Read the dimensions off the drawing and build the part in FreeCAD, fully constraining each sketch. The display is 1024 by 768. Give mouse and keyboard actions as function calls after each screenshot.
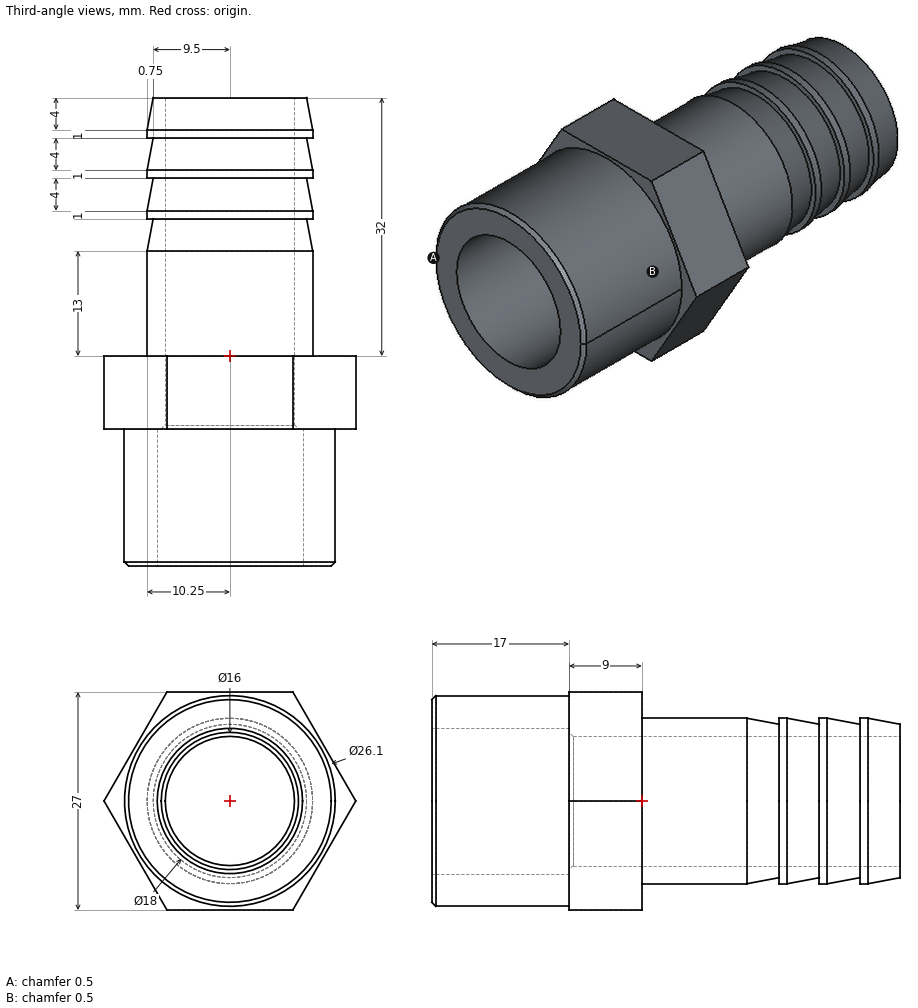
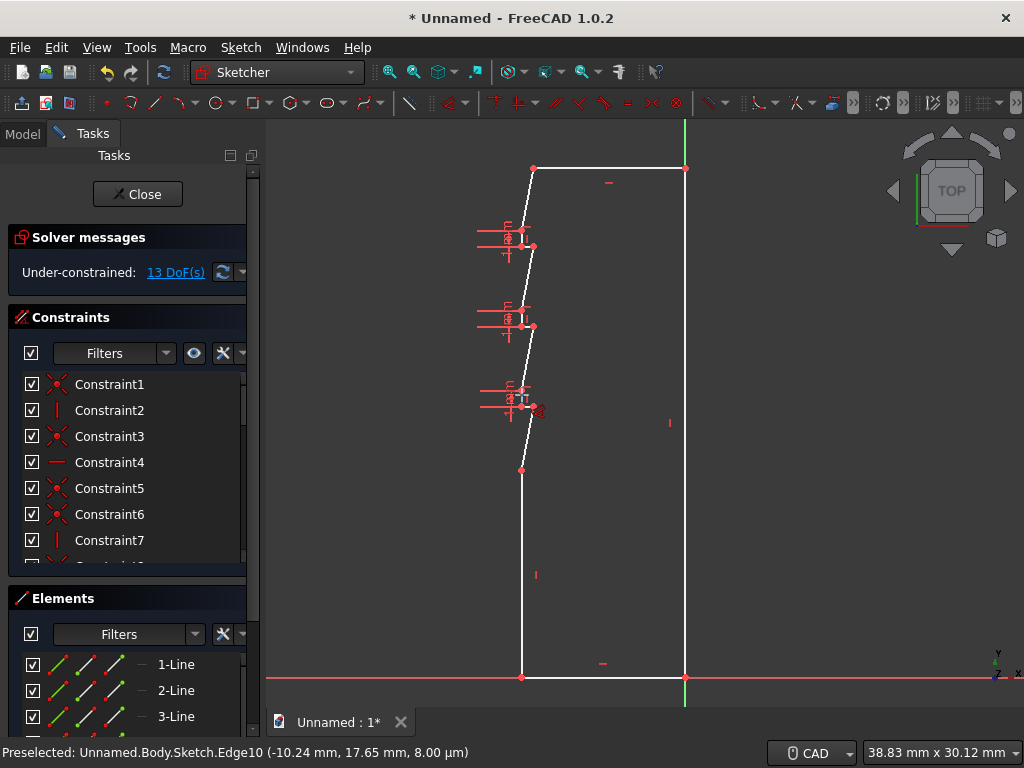
click(631, 482)
click(665, 414)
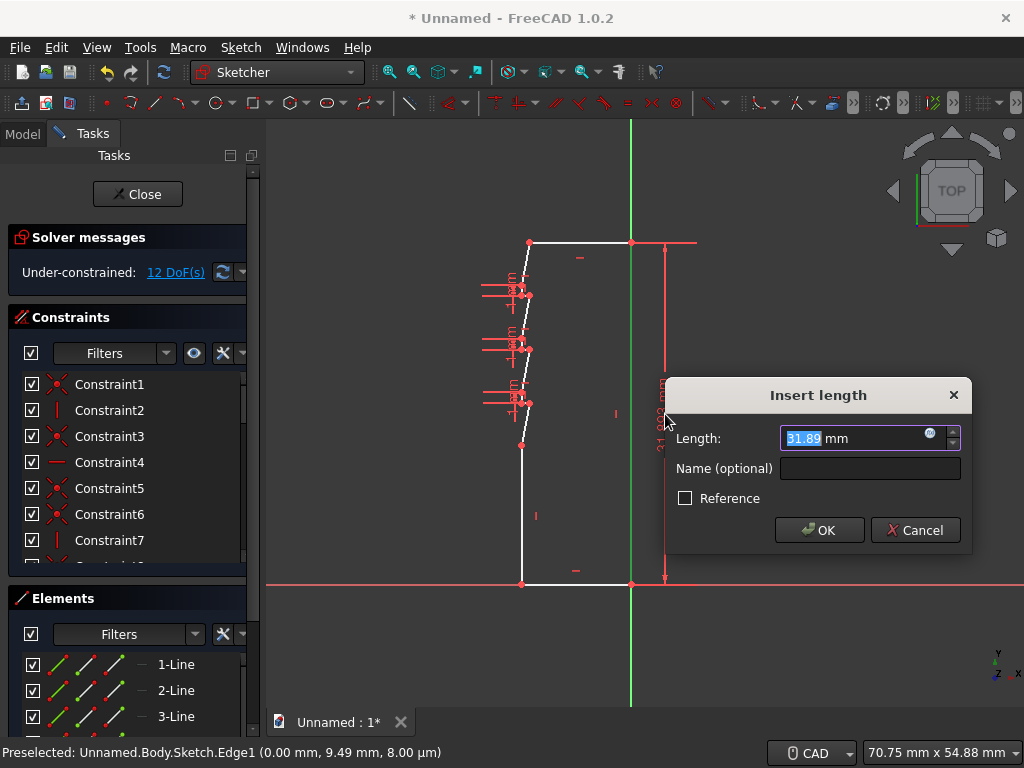
text(32)
key(Return)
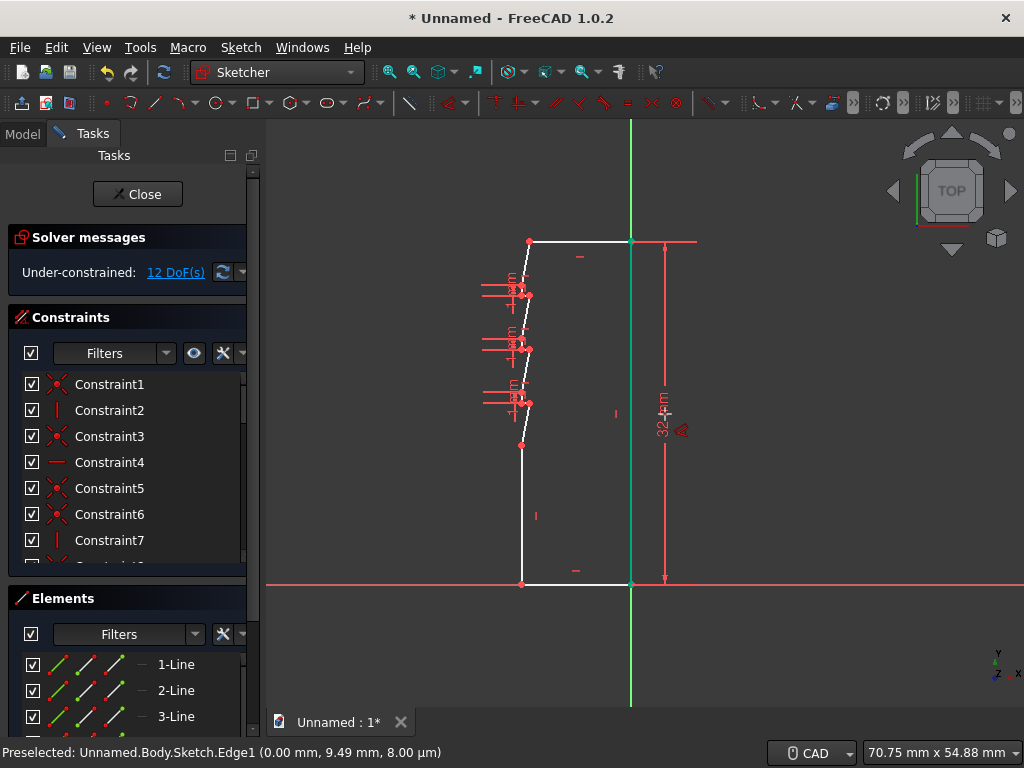
click(522, 487)
click(488, 515)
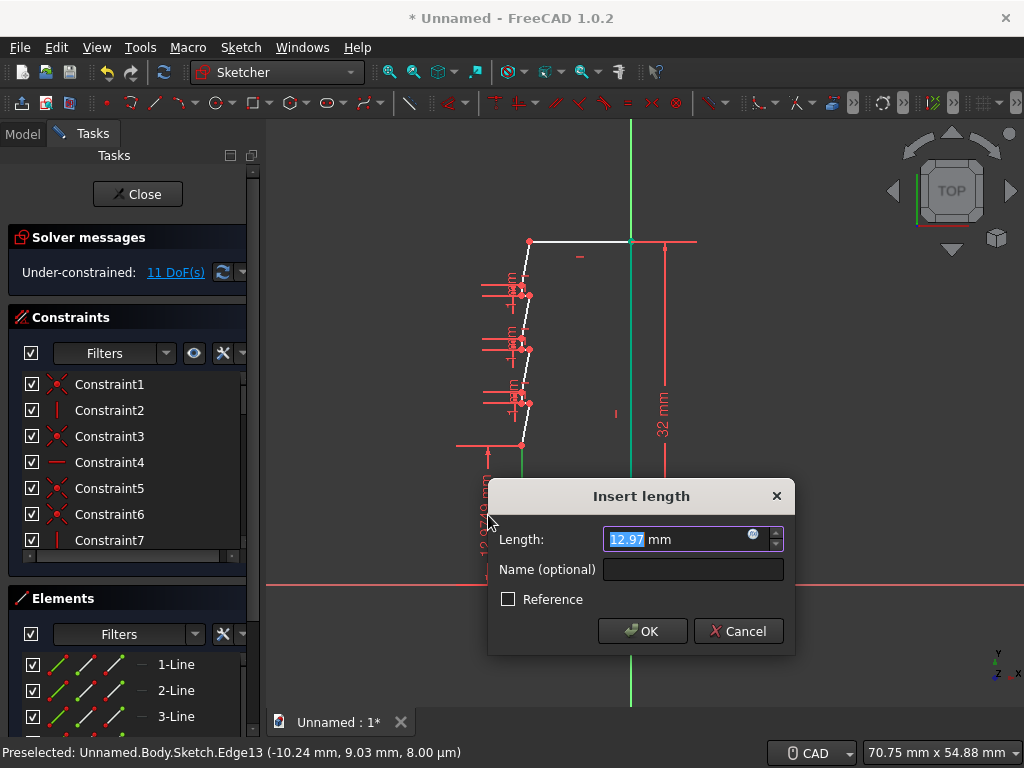
text(13)
key(Return)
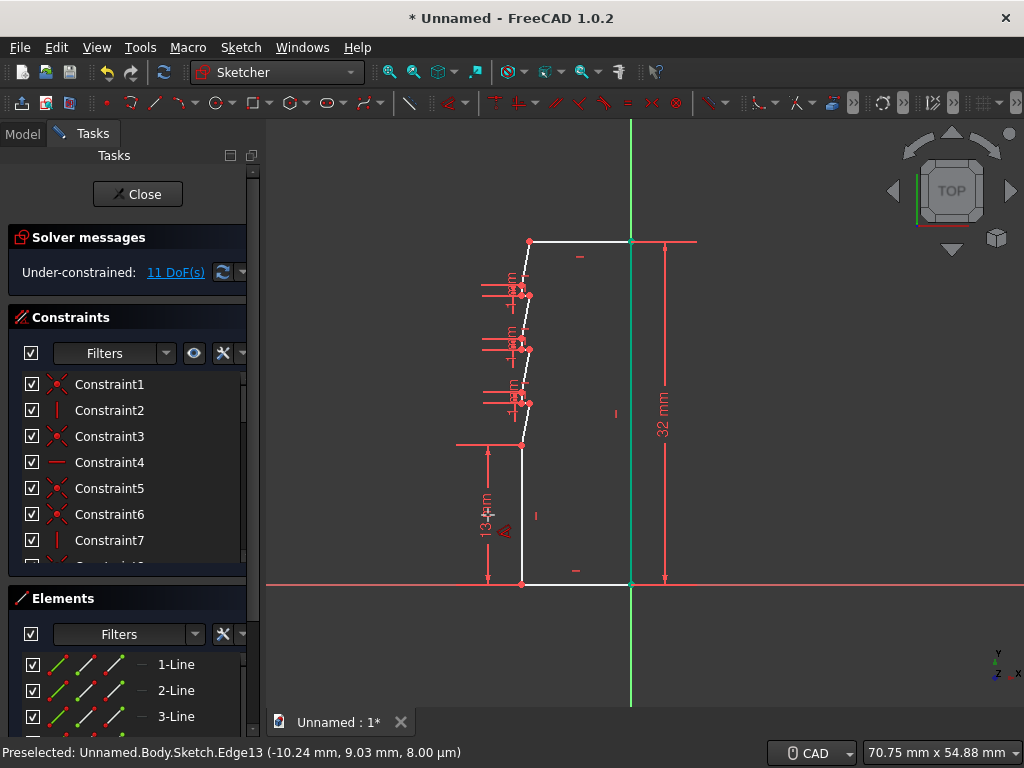
click(527, 255)
click(488, 263)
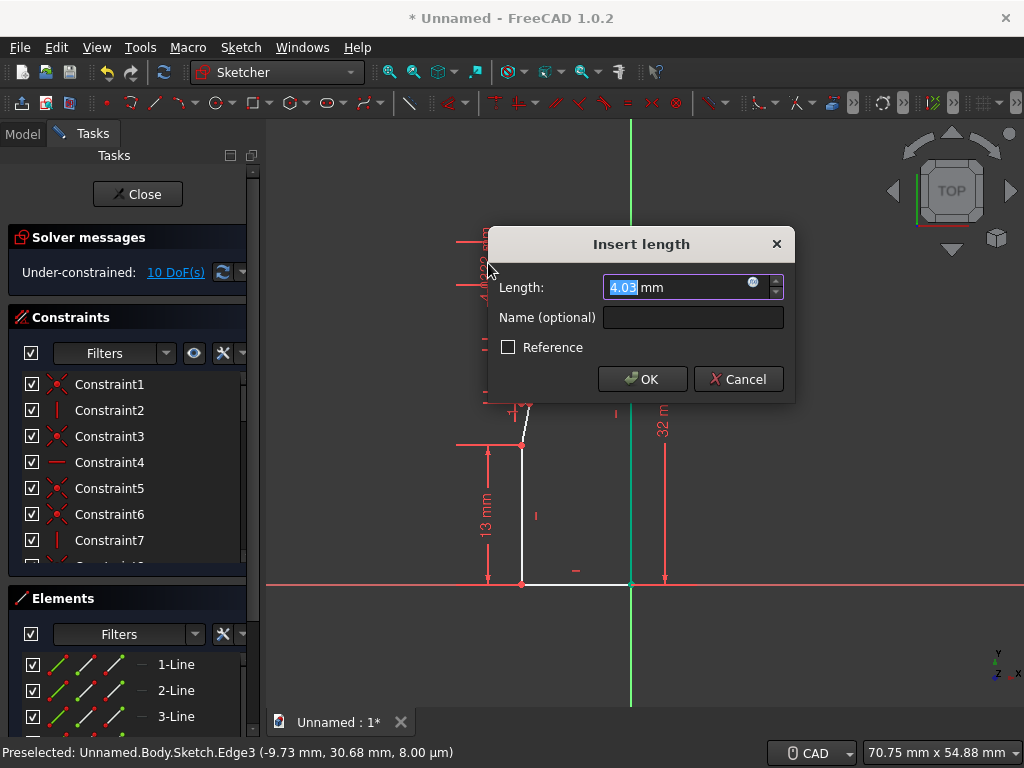
text(4)
key(Return)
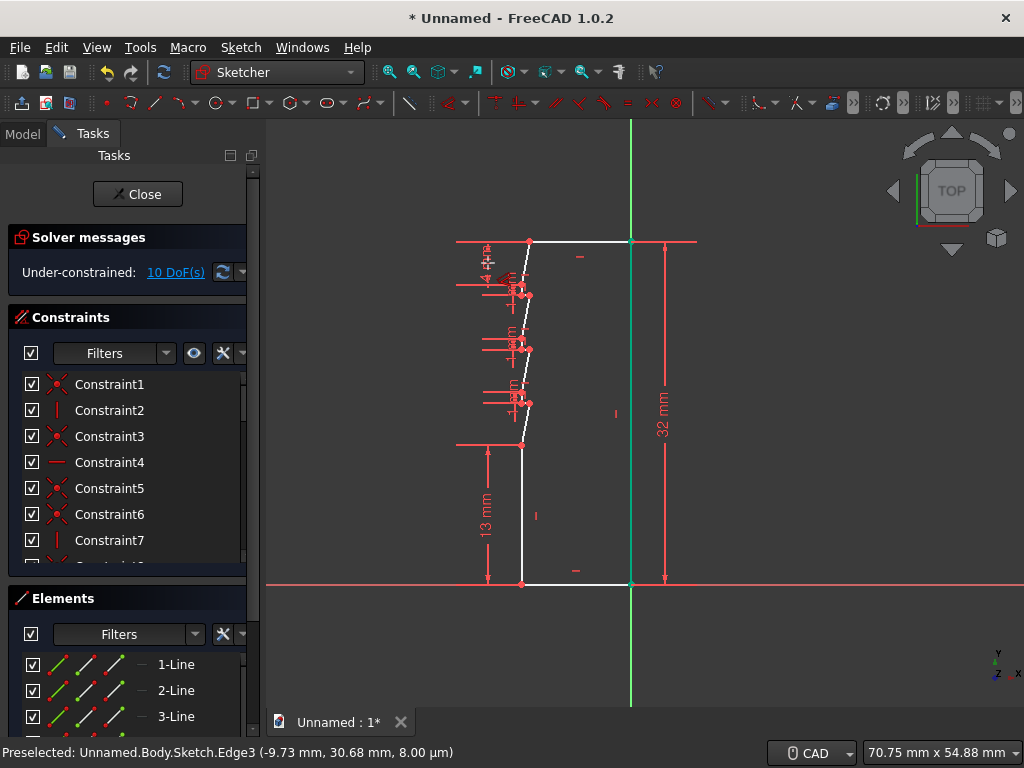
click(527, 308)
click(488, 317)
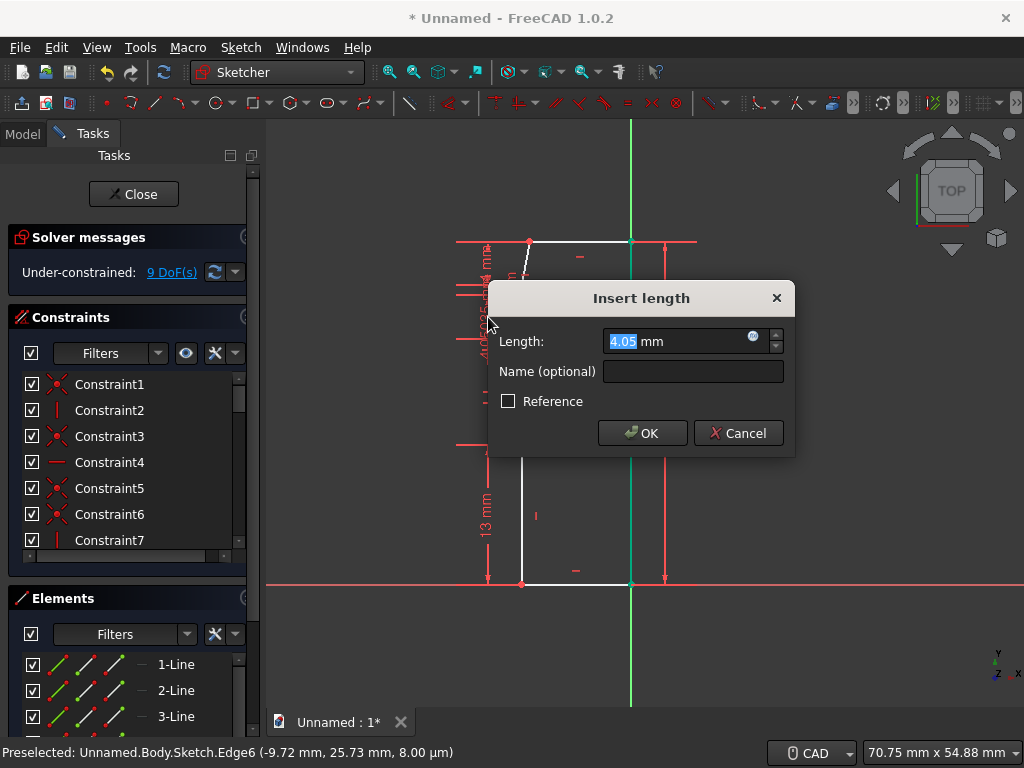
text(4)
key(Return)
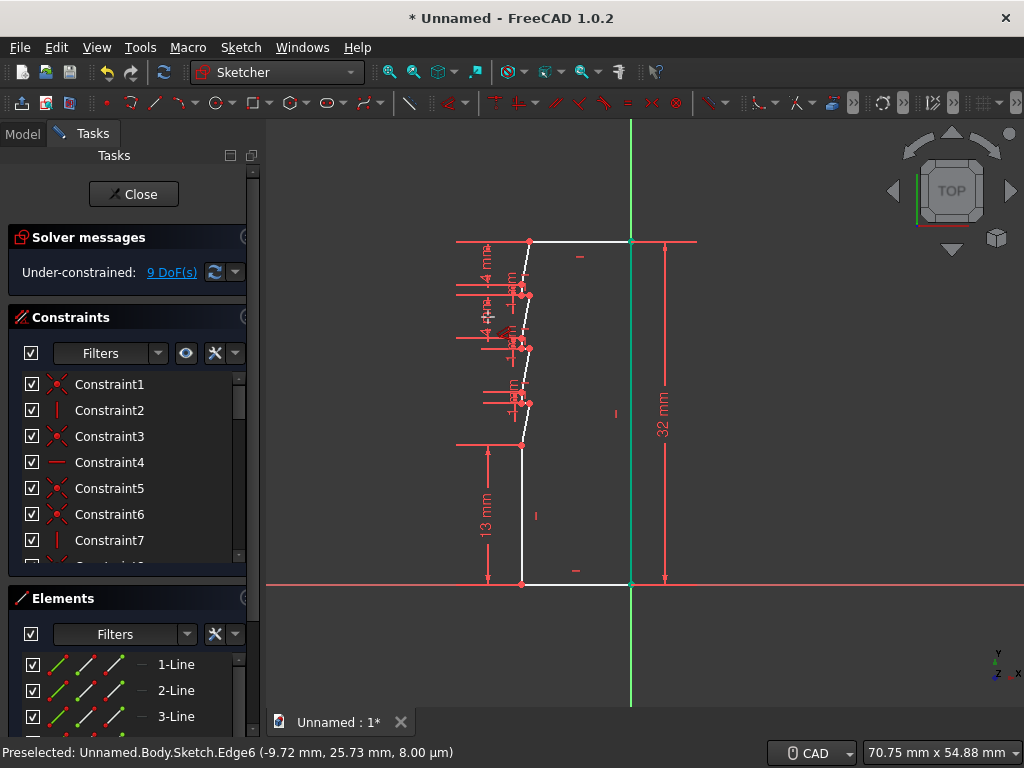
click(527, 362)
click(488, 371)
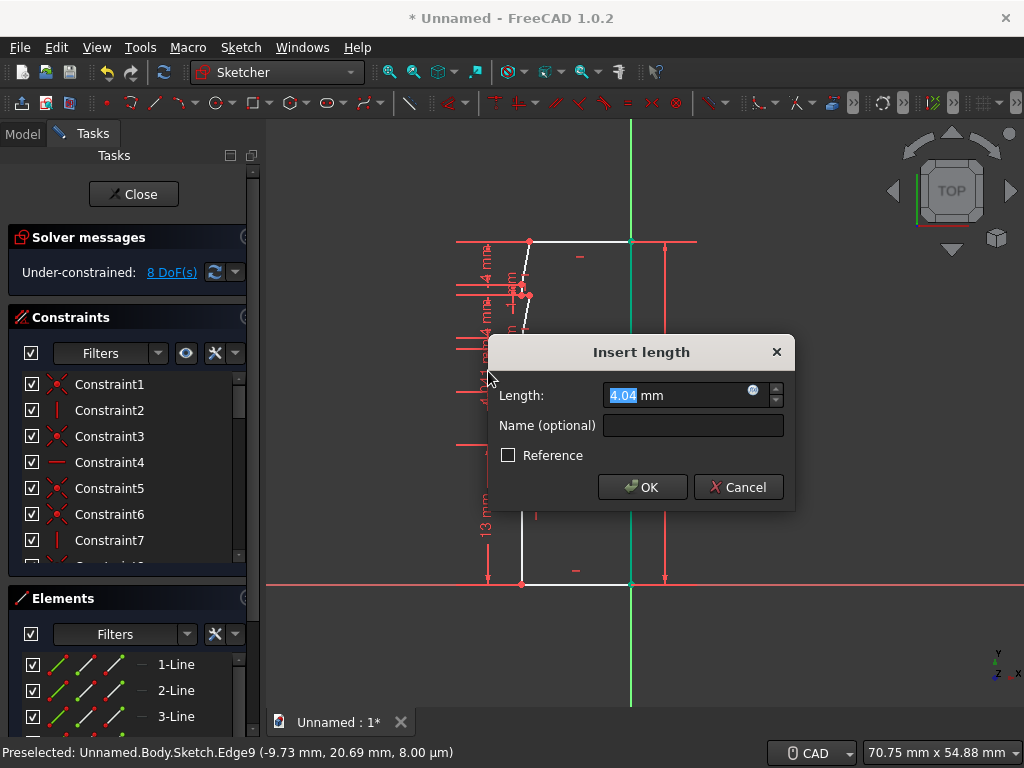
text(4)
key(Return)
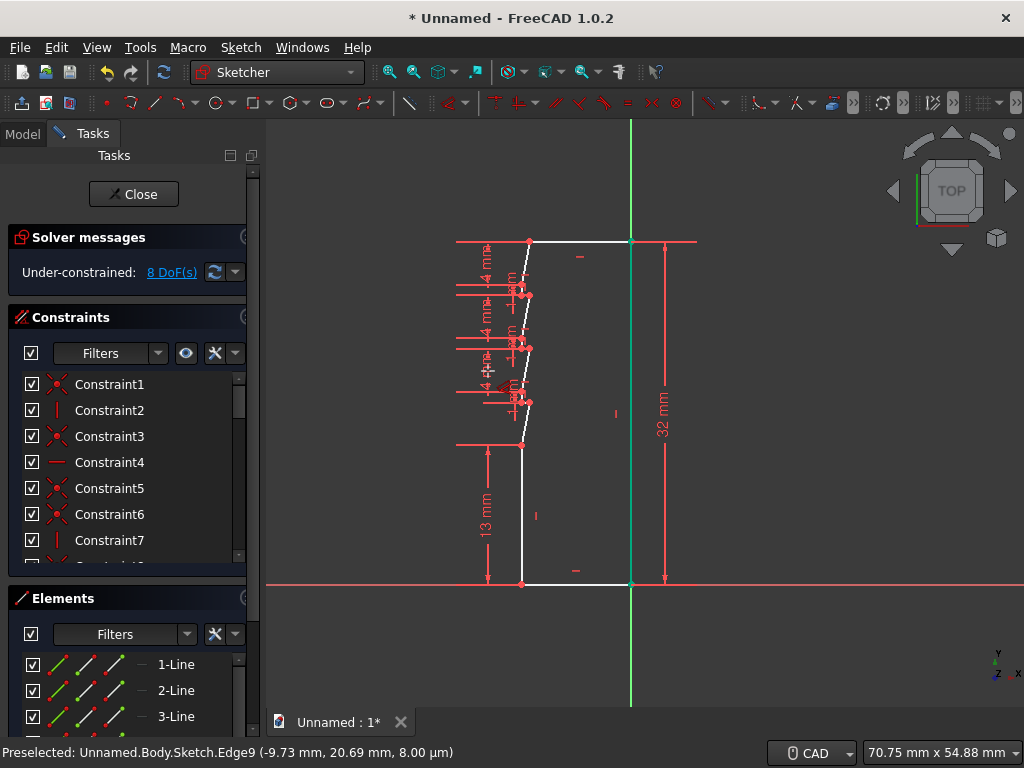
click(601, 242)
click(581, 208)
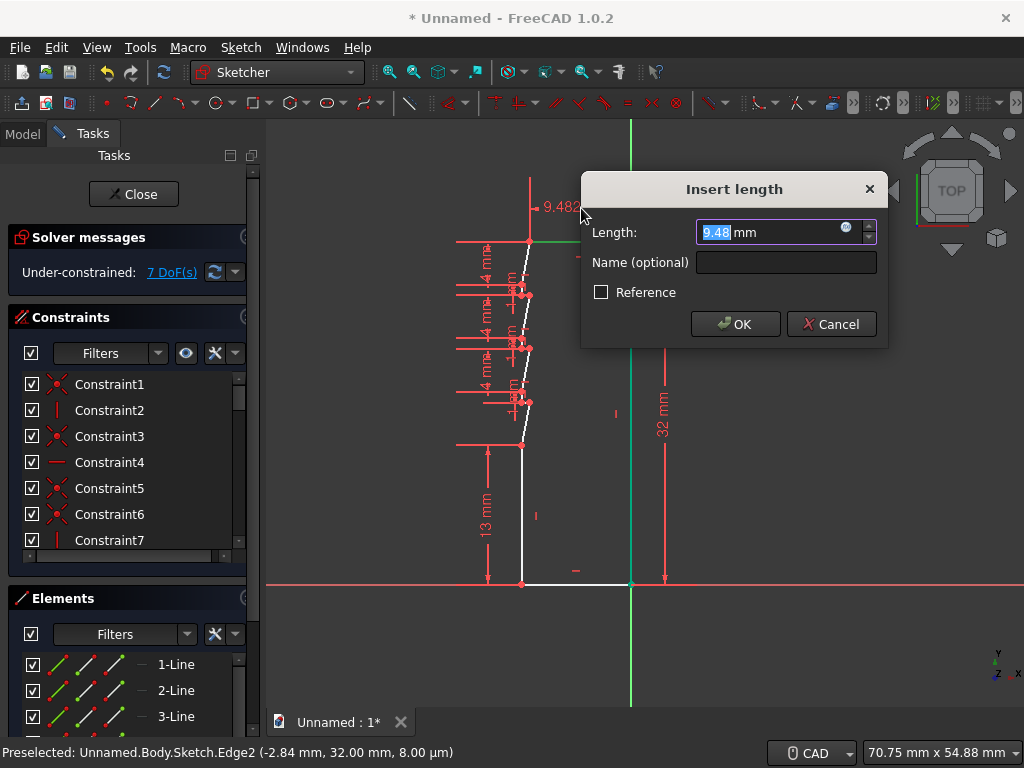
text(9.5)
key(Return)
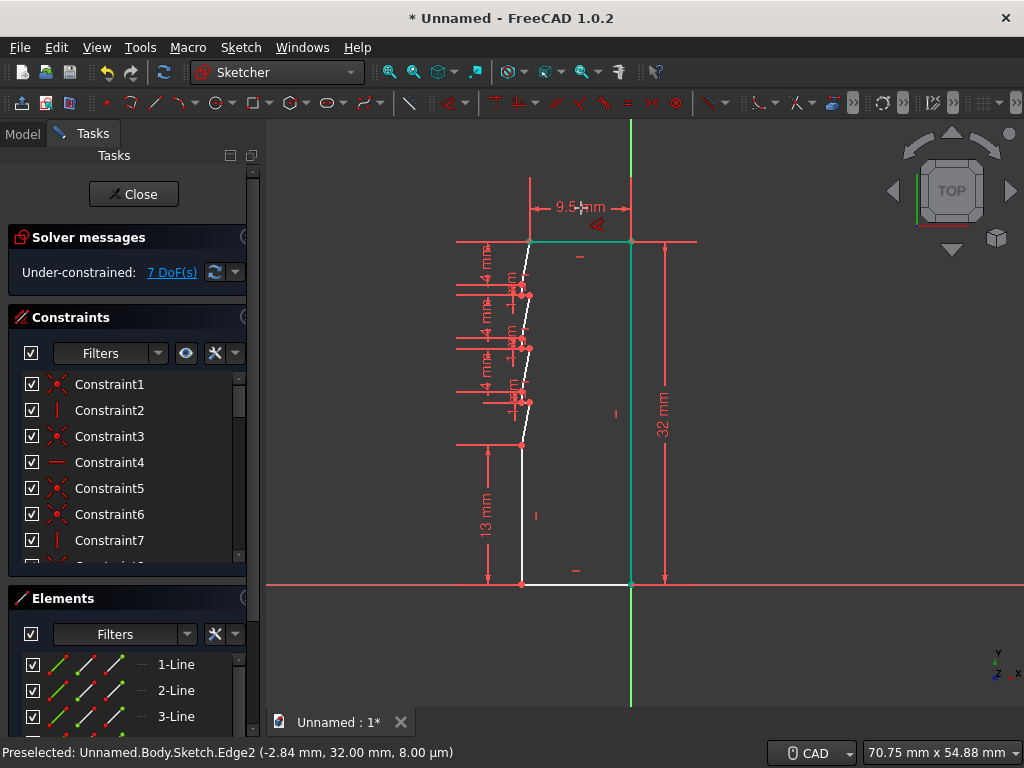
scroll(526, 295, up, 8)